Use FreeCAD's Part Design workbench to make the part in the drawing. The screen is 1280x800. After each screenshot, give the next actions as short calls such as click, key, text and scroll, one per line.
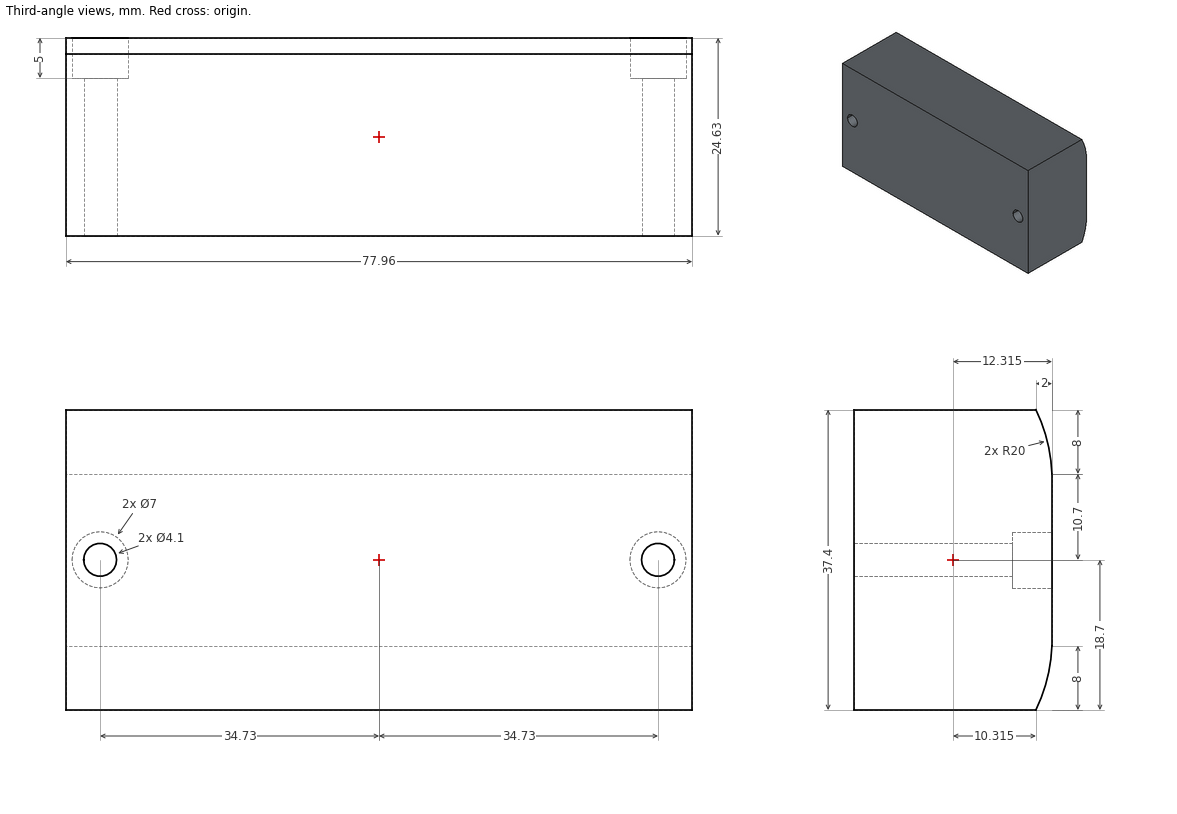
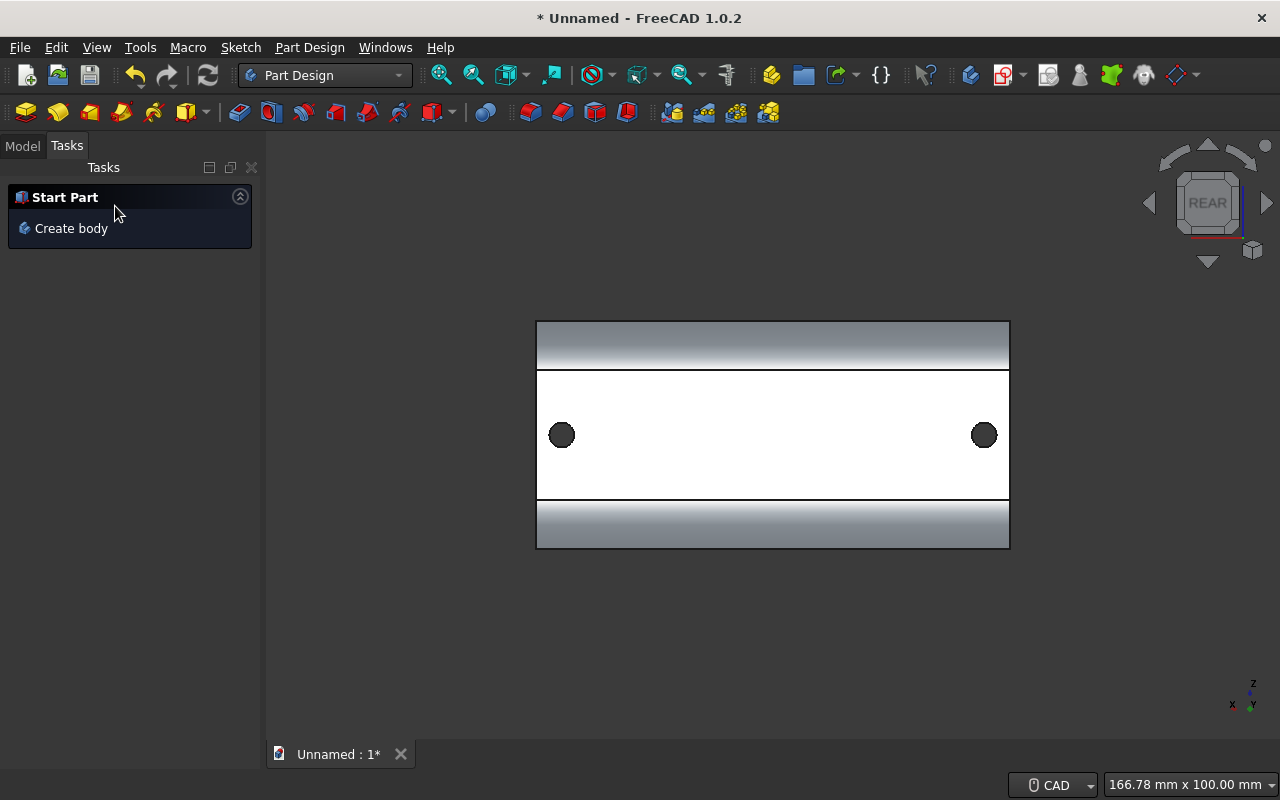
click(705, 434)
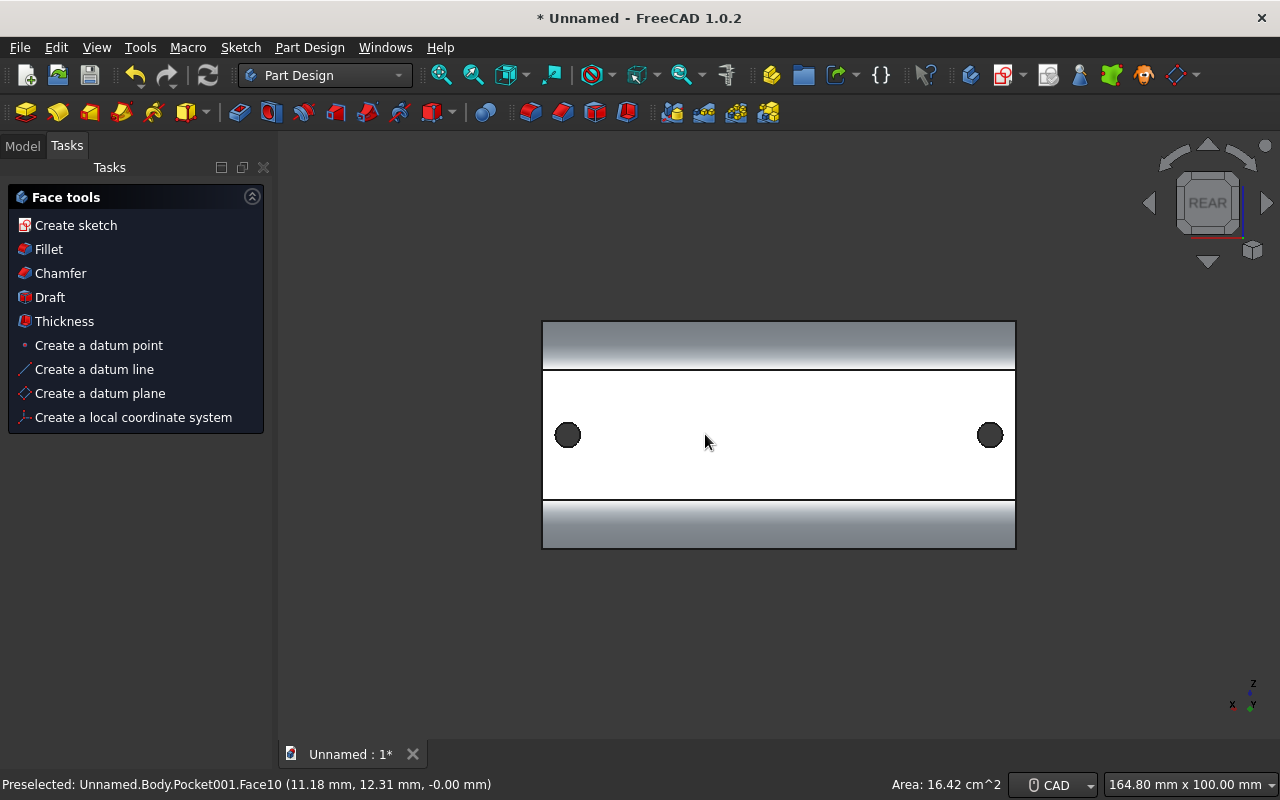
click(1004, 76)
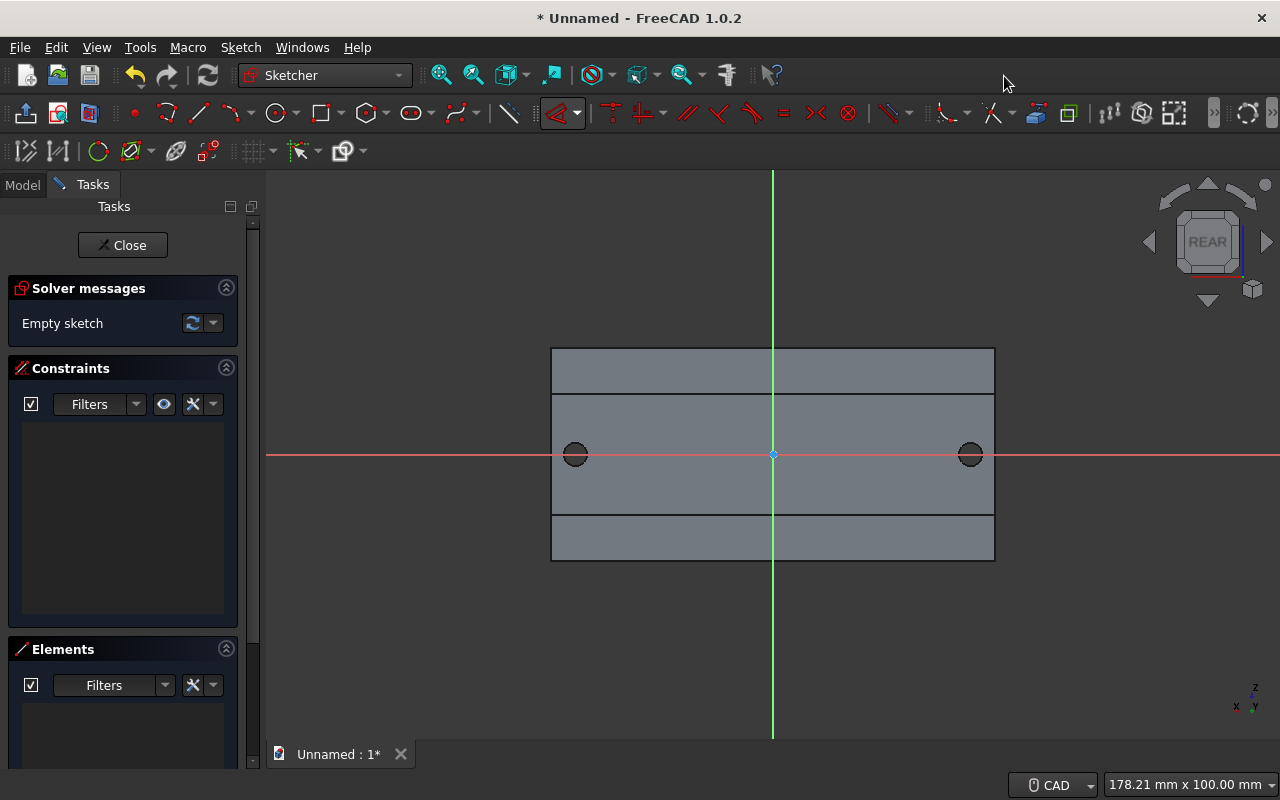
click(276, 114)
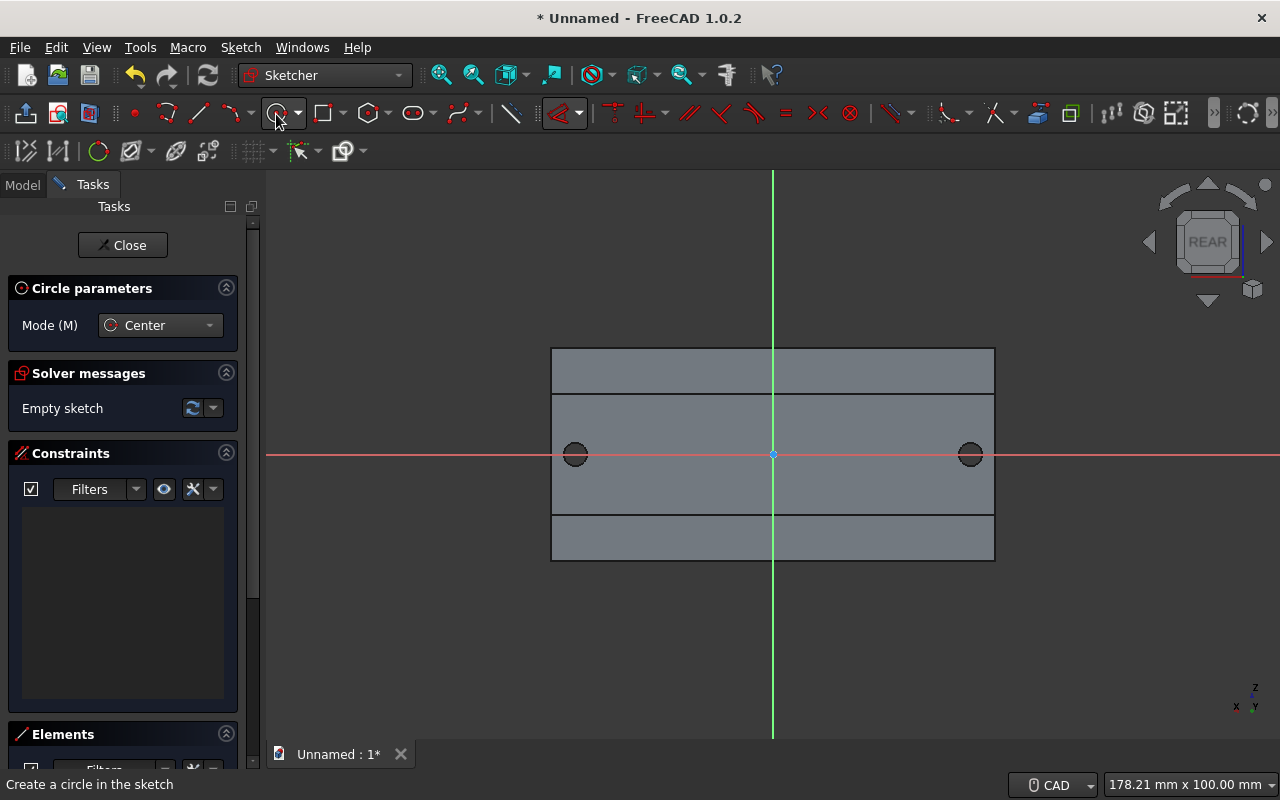
click(971, 455)
click(985, 440)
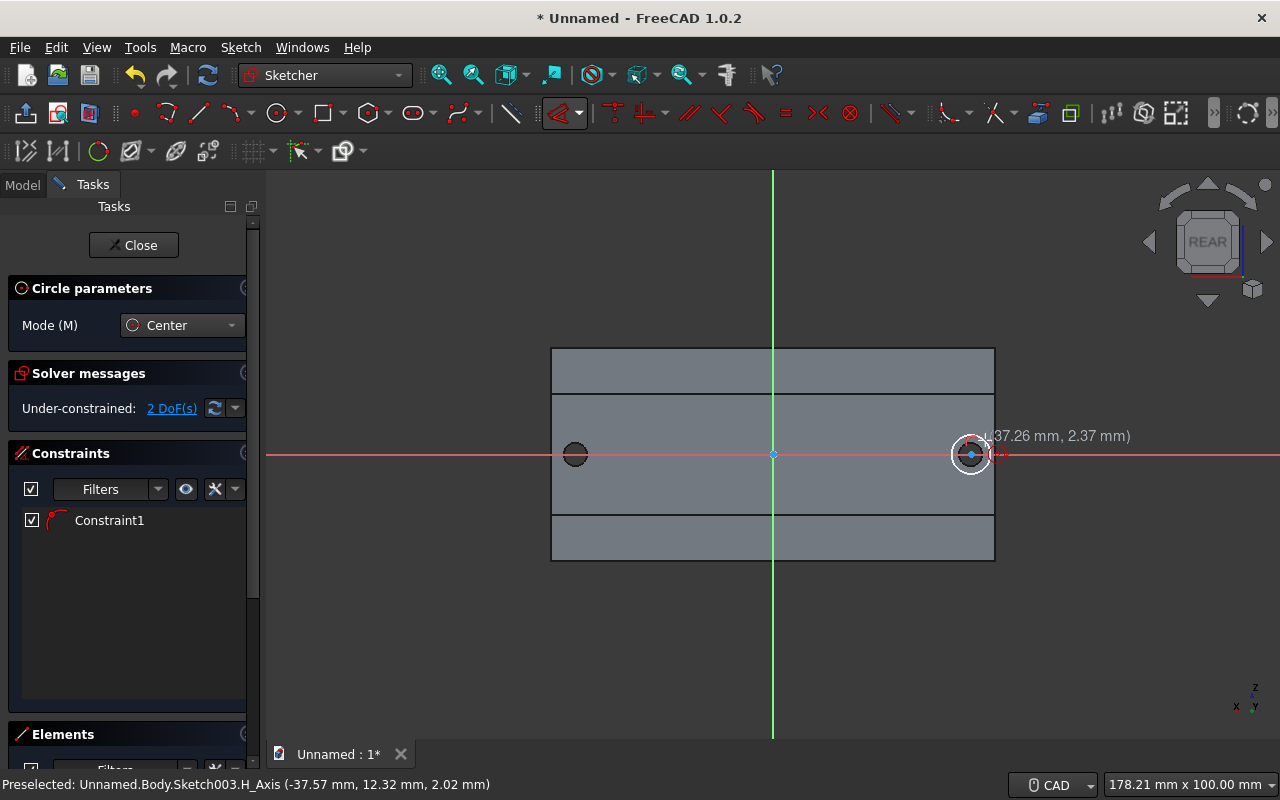
click(575, 455)
click(589, 440)
key(Escape)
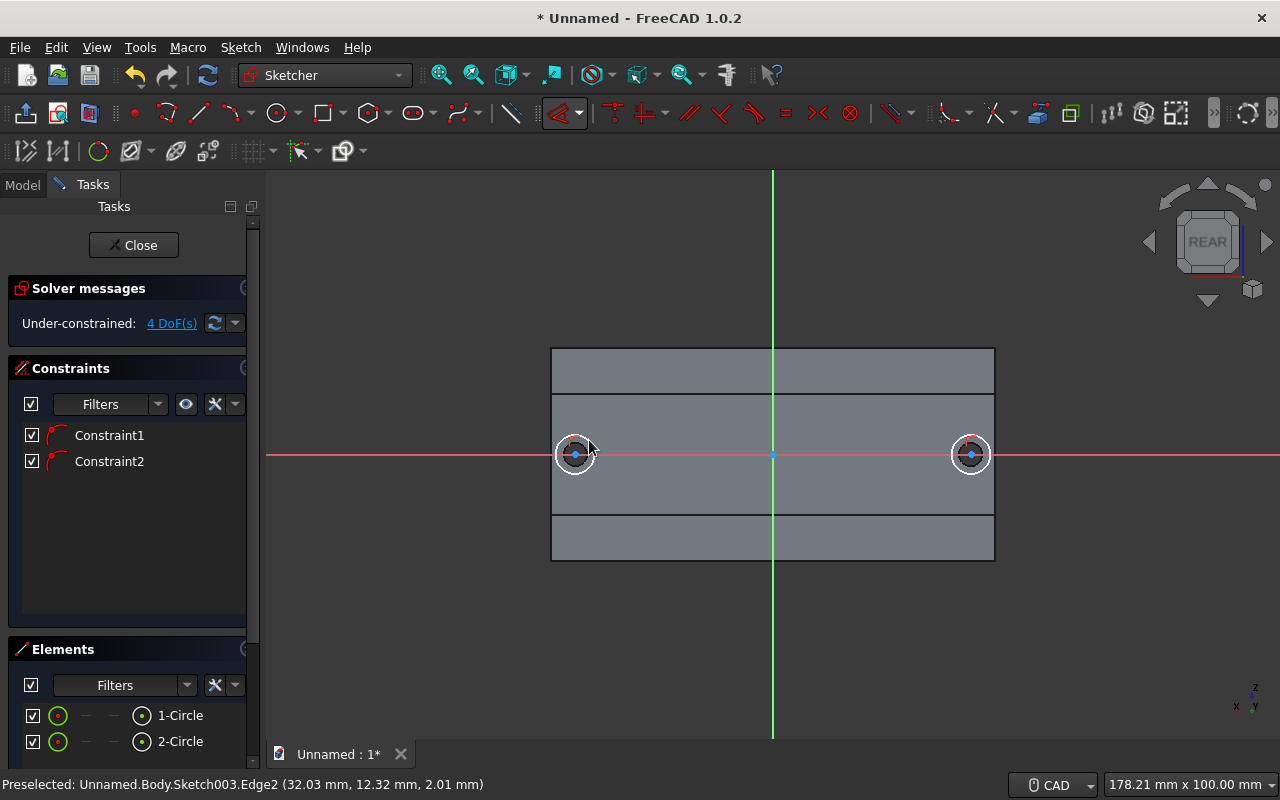
click(985, 441)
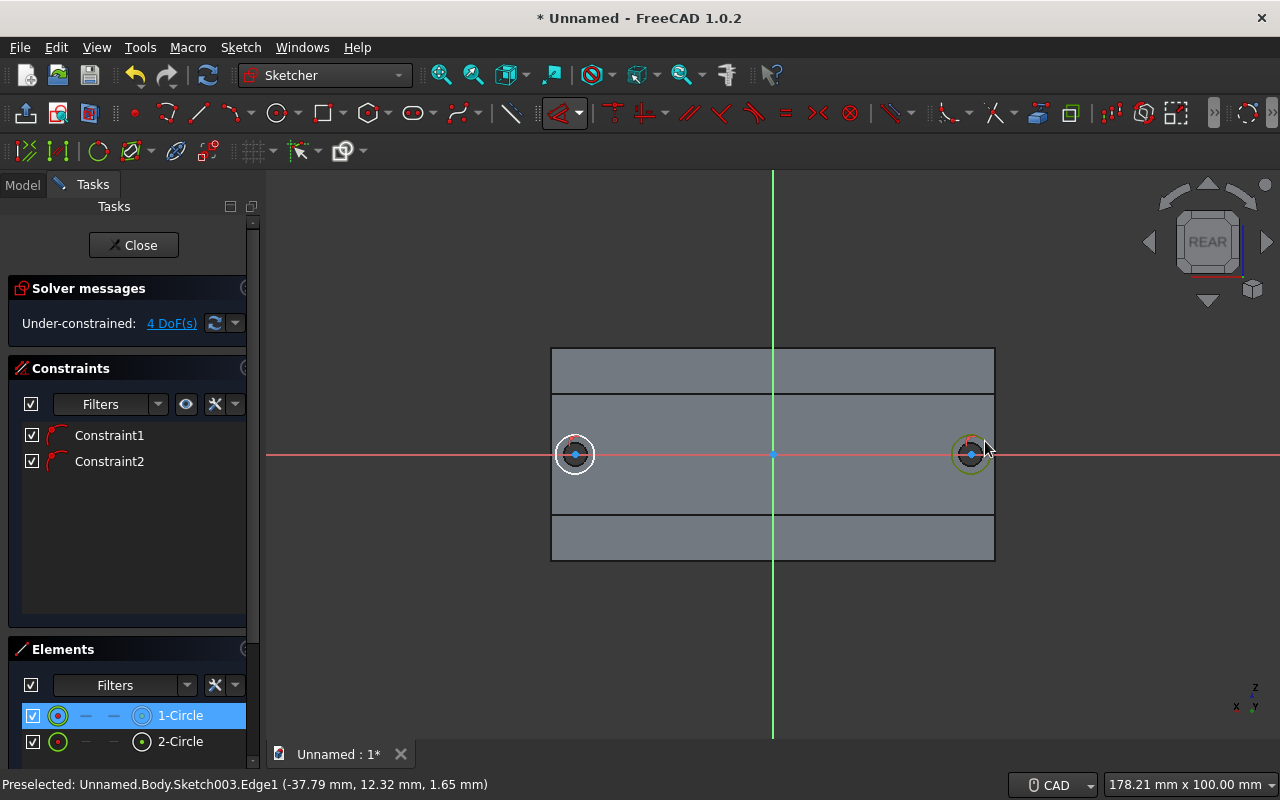
click(589, 441)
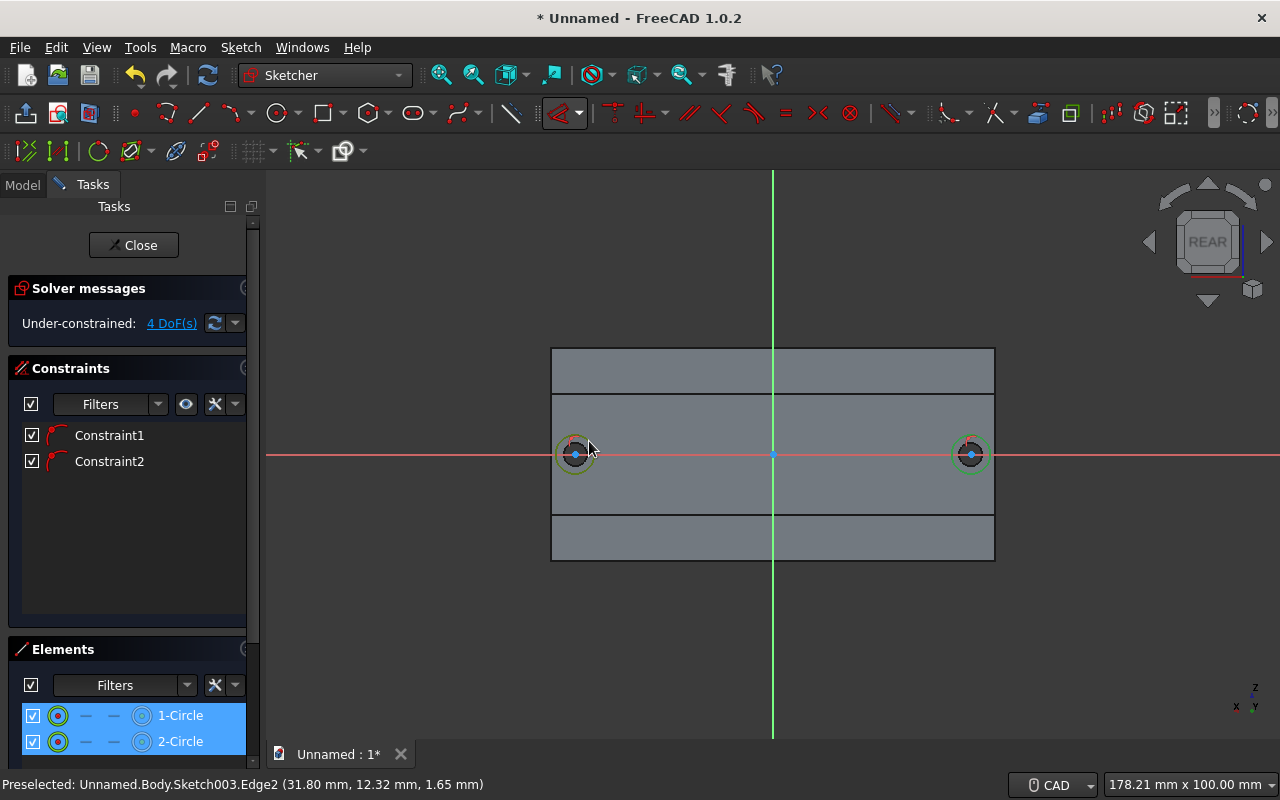
click(786, 114)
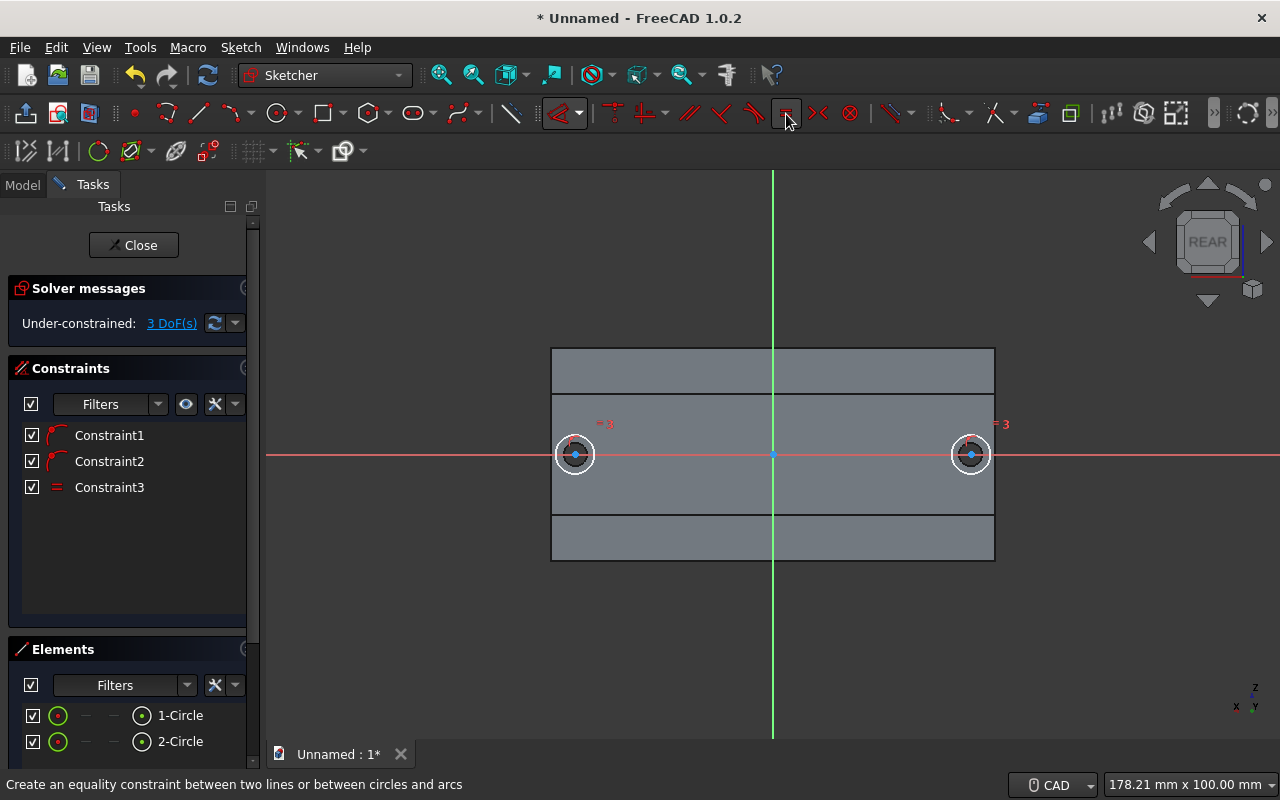
click(985, 441)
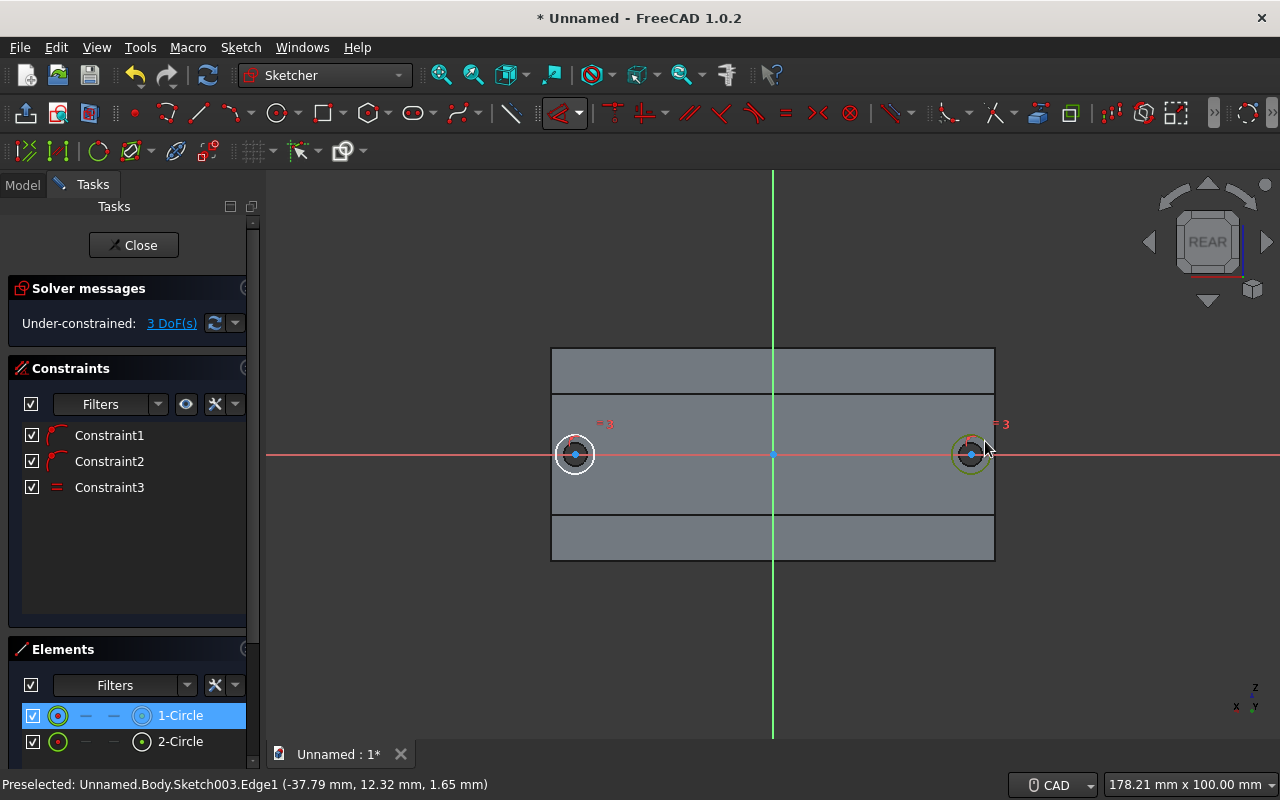
key(k)
key(o)